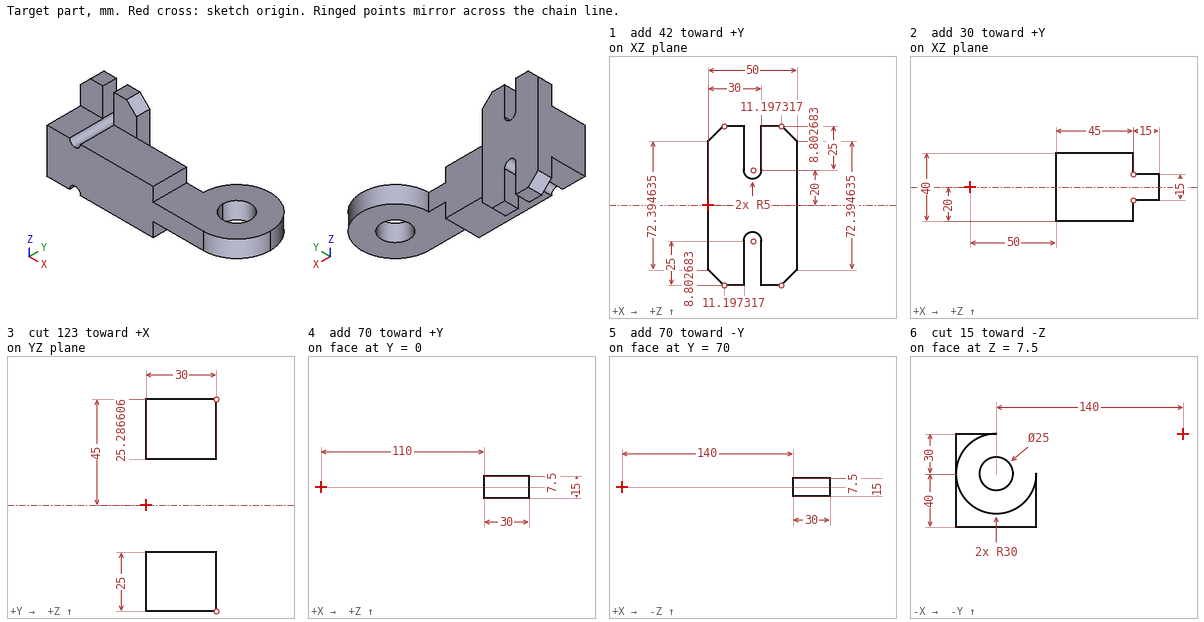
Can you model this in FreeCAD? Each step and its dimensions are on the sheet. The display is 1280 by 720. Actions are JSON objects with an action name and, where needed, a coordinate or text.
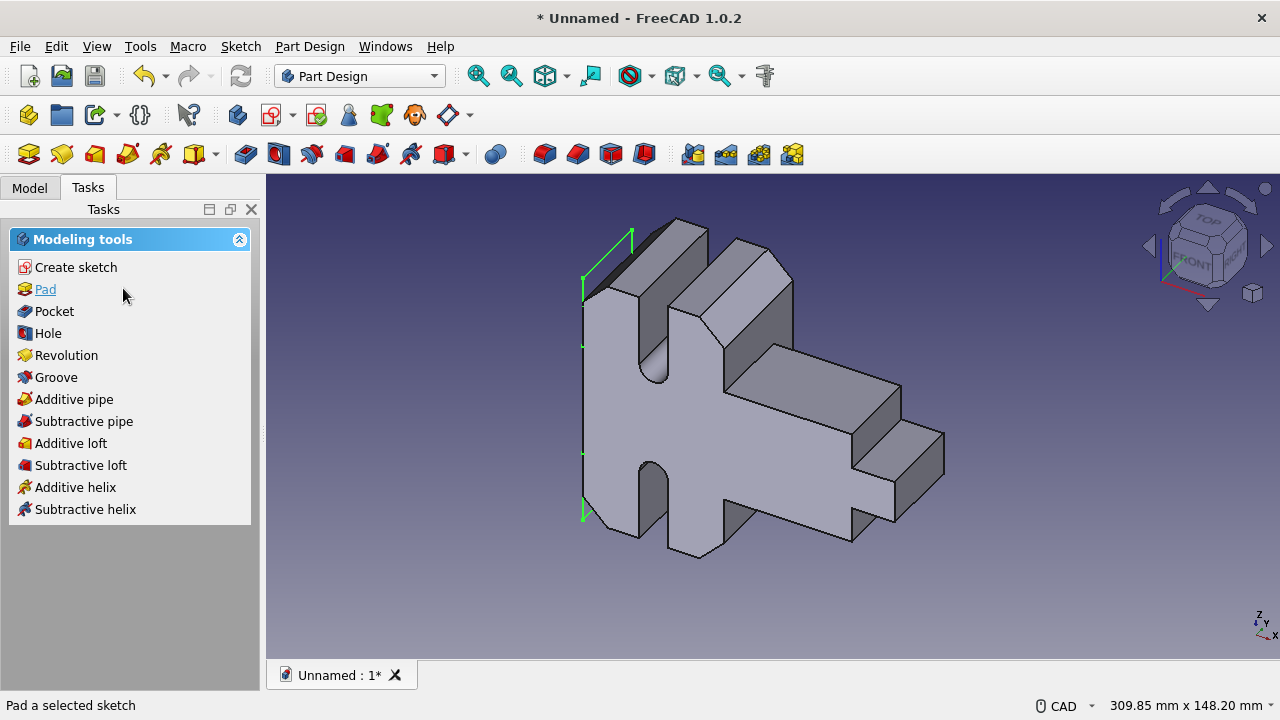
{"action": "left_click", "coordinate": [246, 154]}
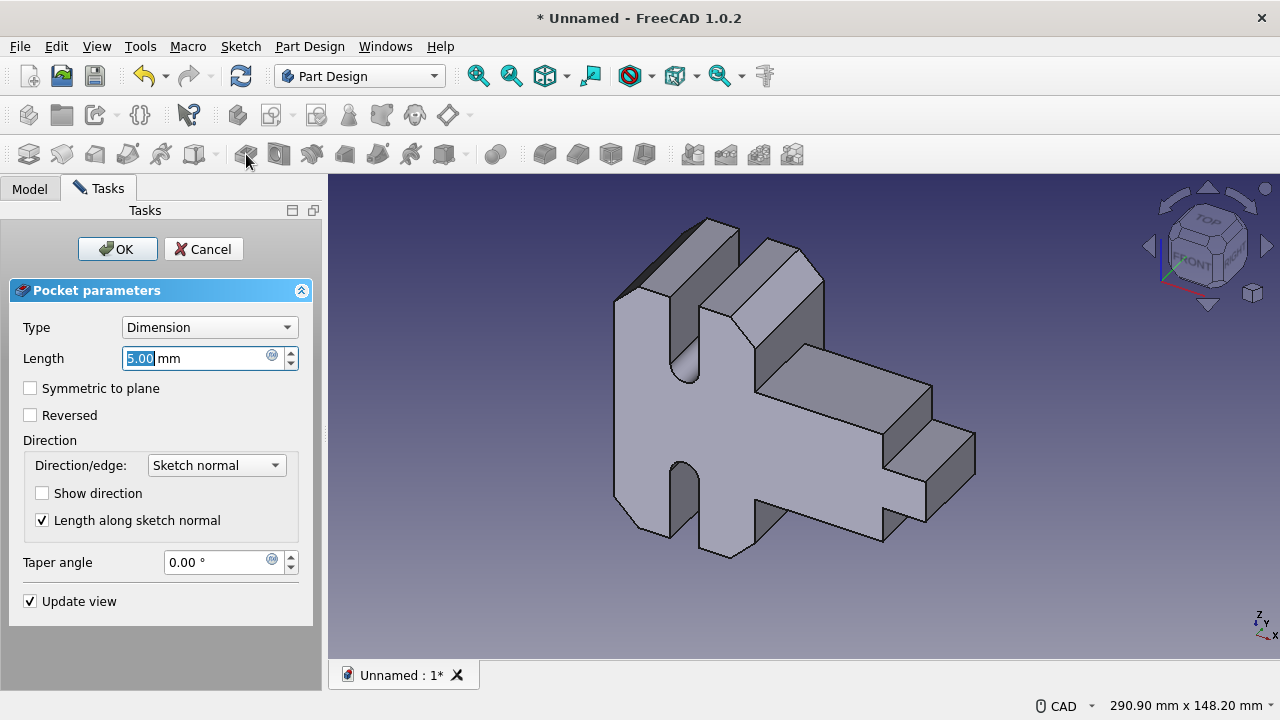
{"action": "type", "text": "123"}
{"action": "key", "text": "Tab"}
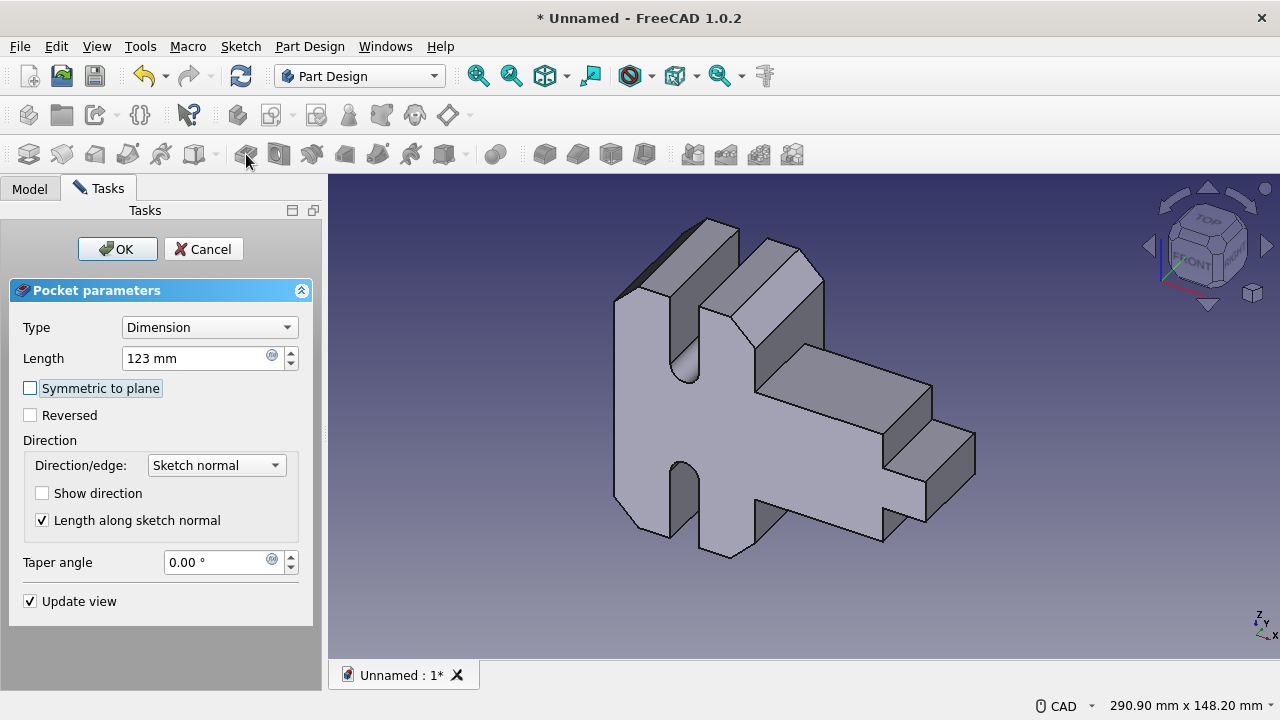
{"action": "left_click", "coordinate": [31, 415]}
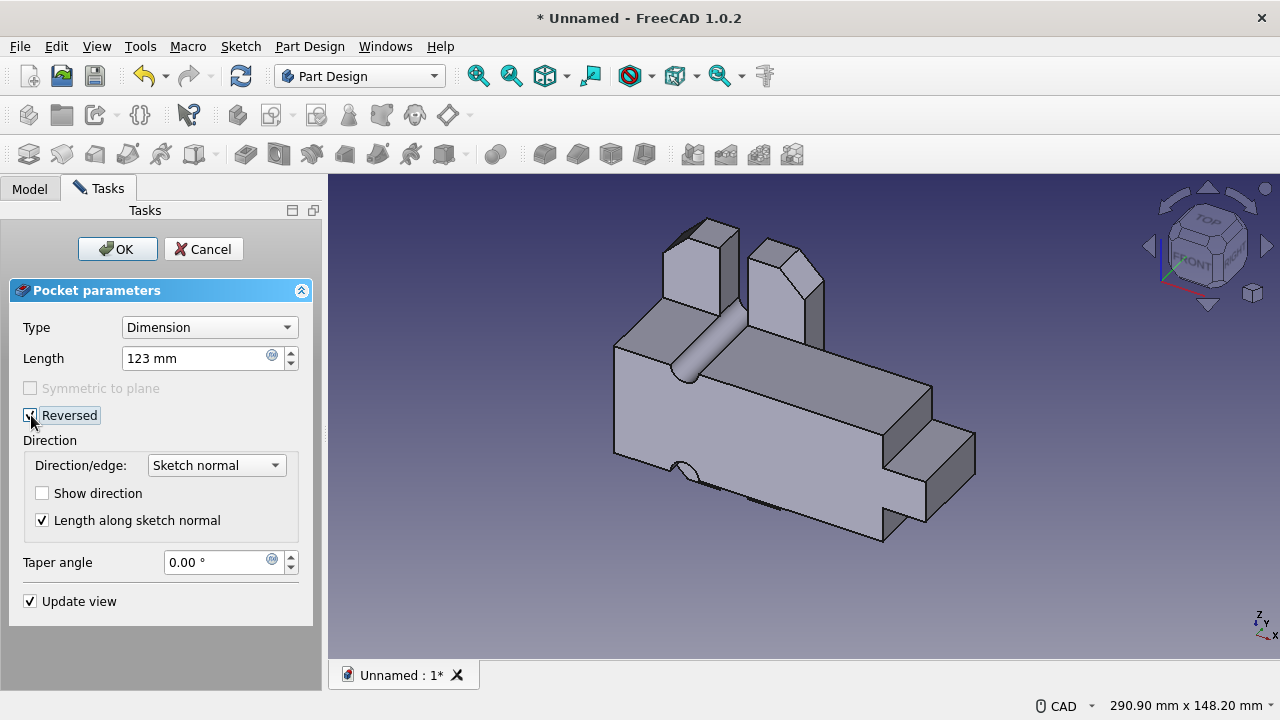
{"action": "left_click", "coordinate": [118, 249]}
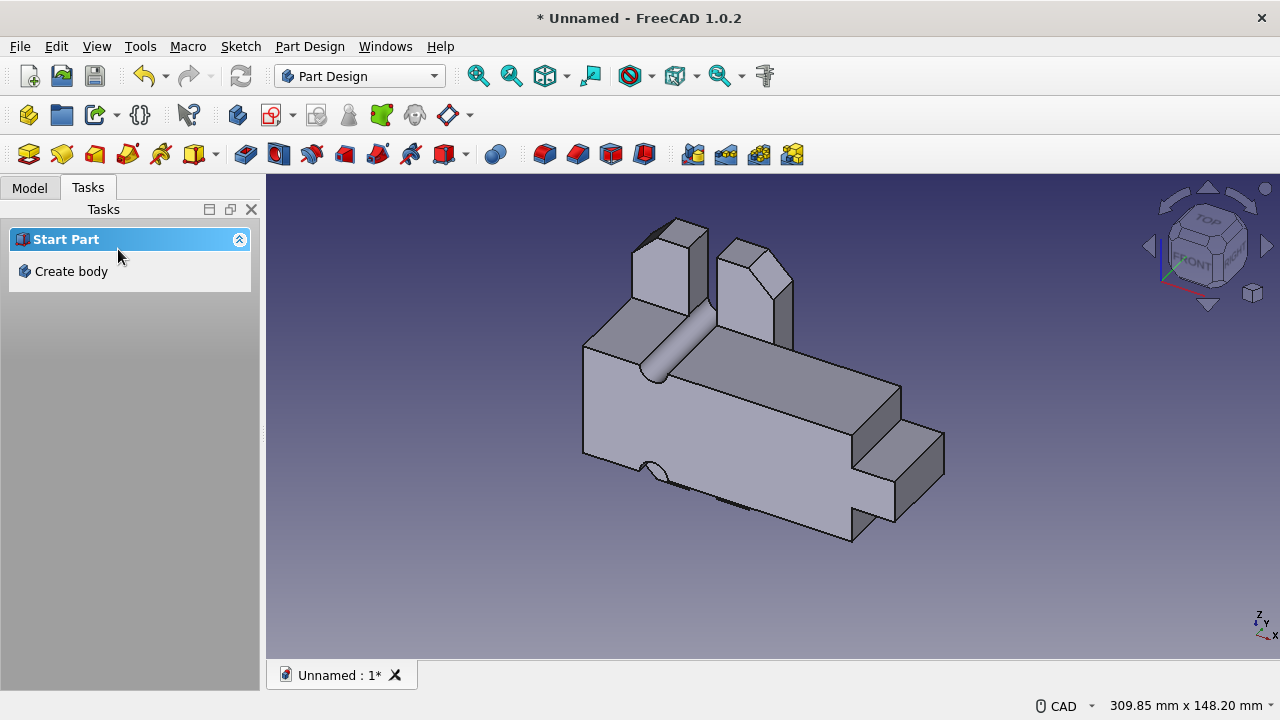
{"action": "left_click", "coordinate": [783, 465]}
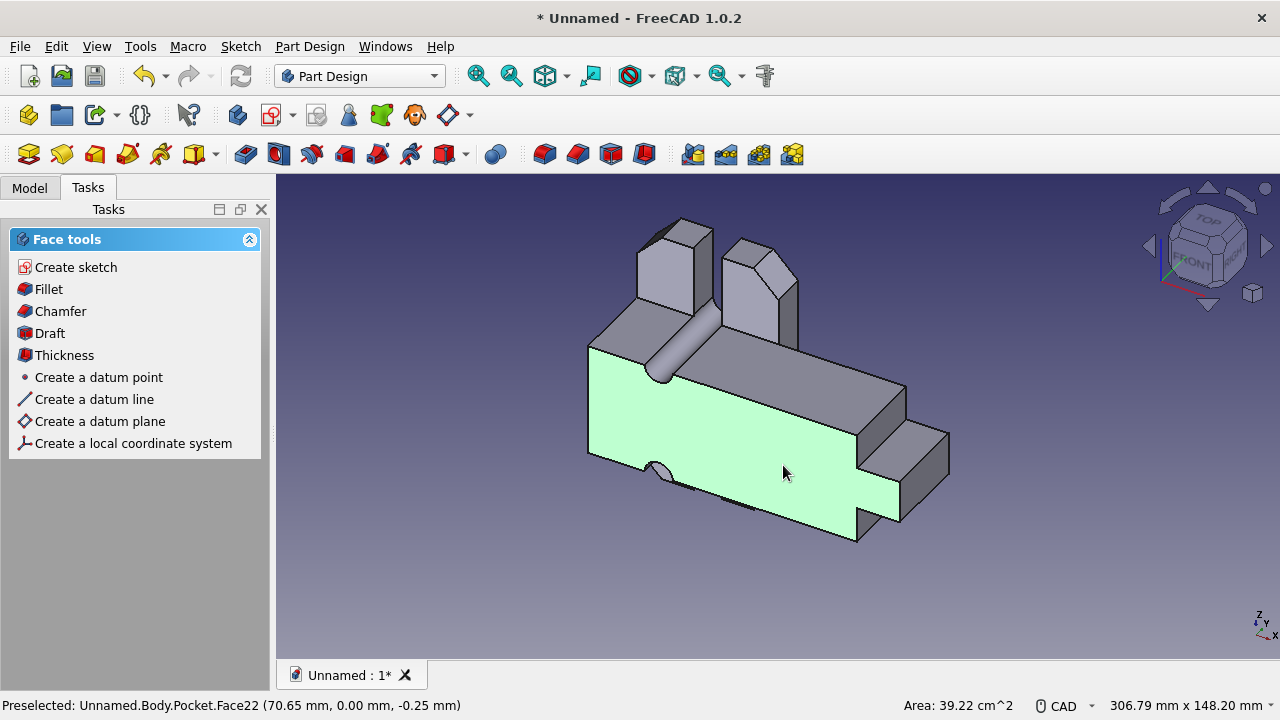
{"action": "left_click", "coordinate": [270, 116]}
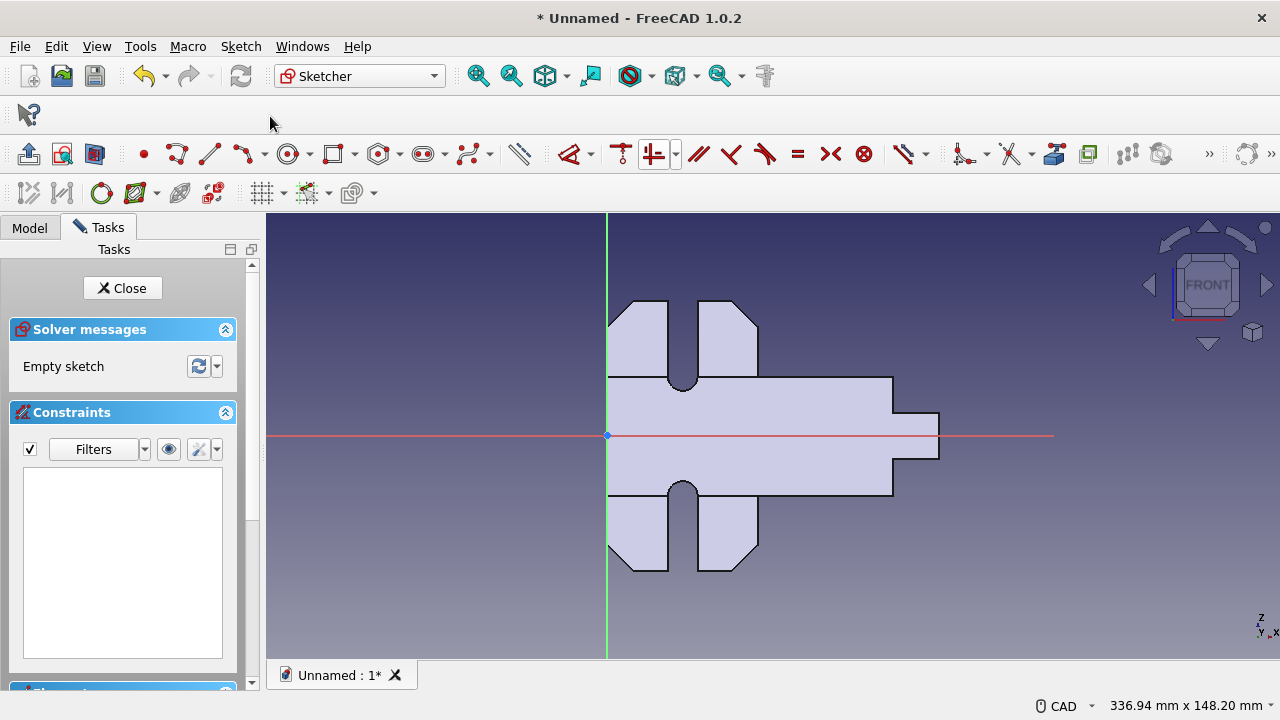
{"action": "scroll", "coordinate": [1039, 436], "scroll_direction": "up", "scroll_amount": 9}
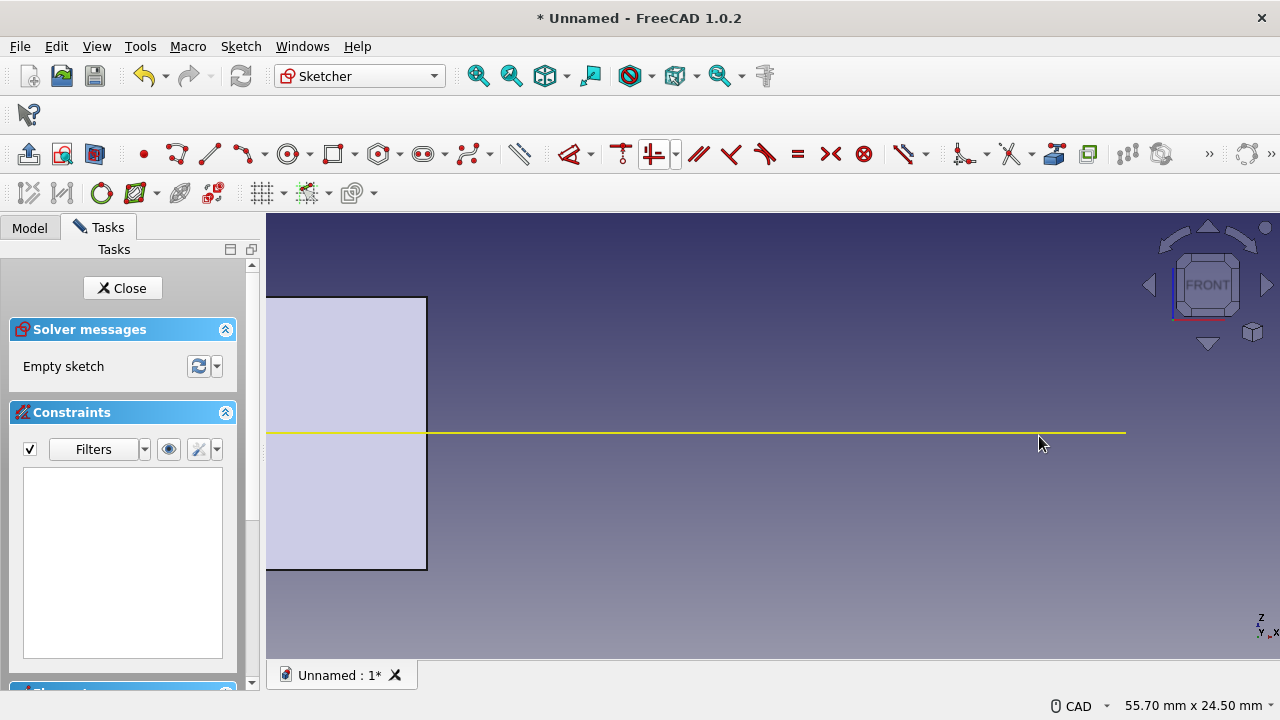
{"action": "left_click", "coordinate": [332, 154]}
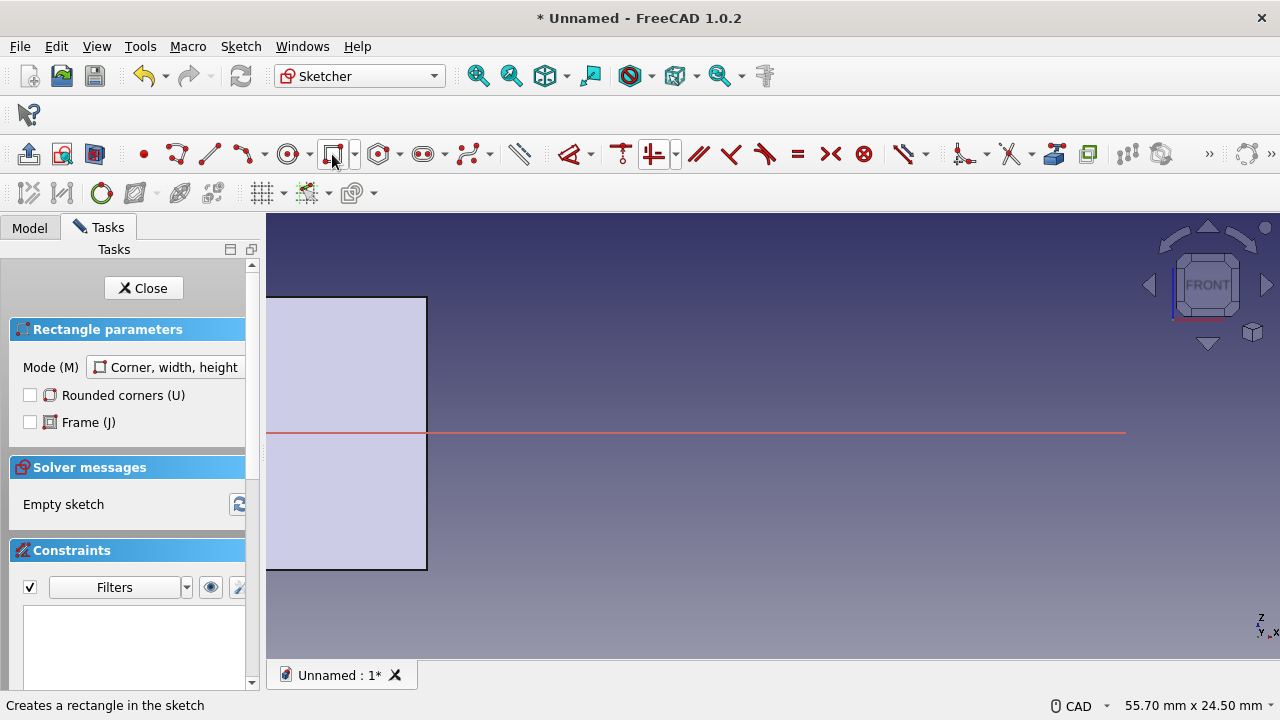
{"action": "left_click", "coordinate": [427, 297]}
{"action": "left_click", "coordinate": [973, 570]}
{"action": "key", "text": "Escape"}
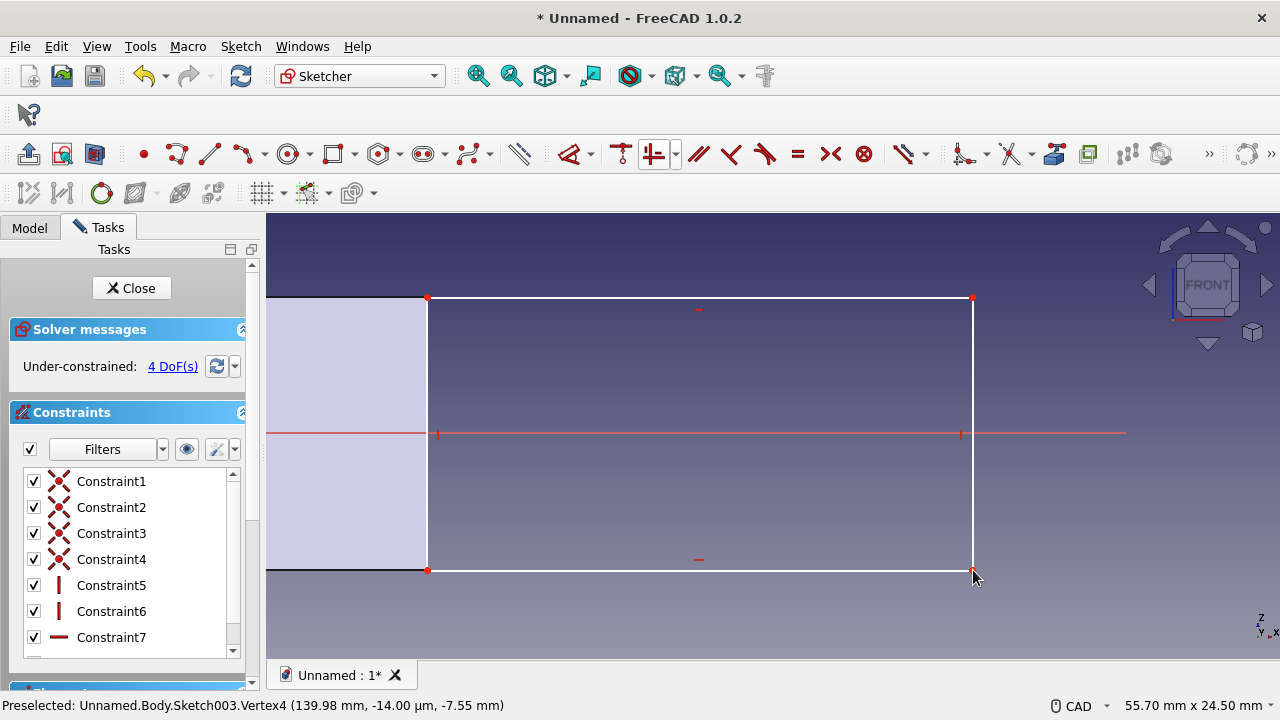
{"action": "left_click", "coordinate": [568, 154]}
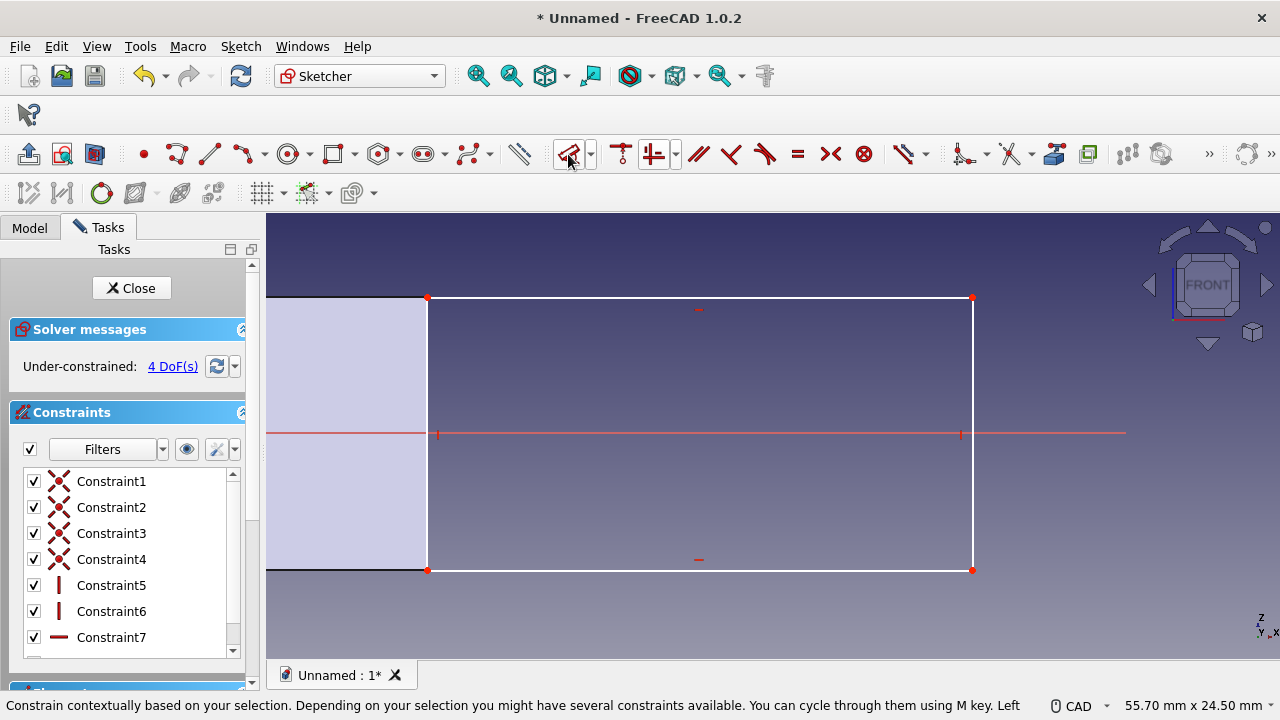
{"action": "left_click", "coordinate": [427, 380]}
{"action": "left_click", "coordinate": [393, 372]}